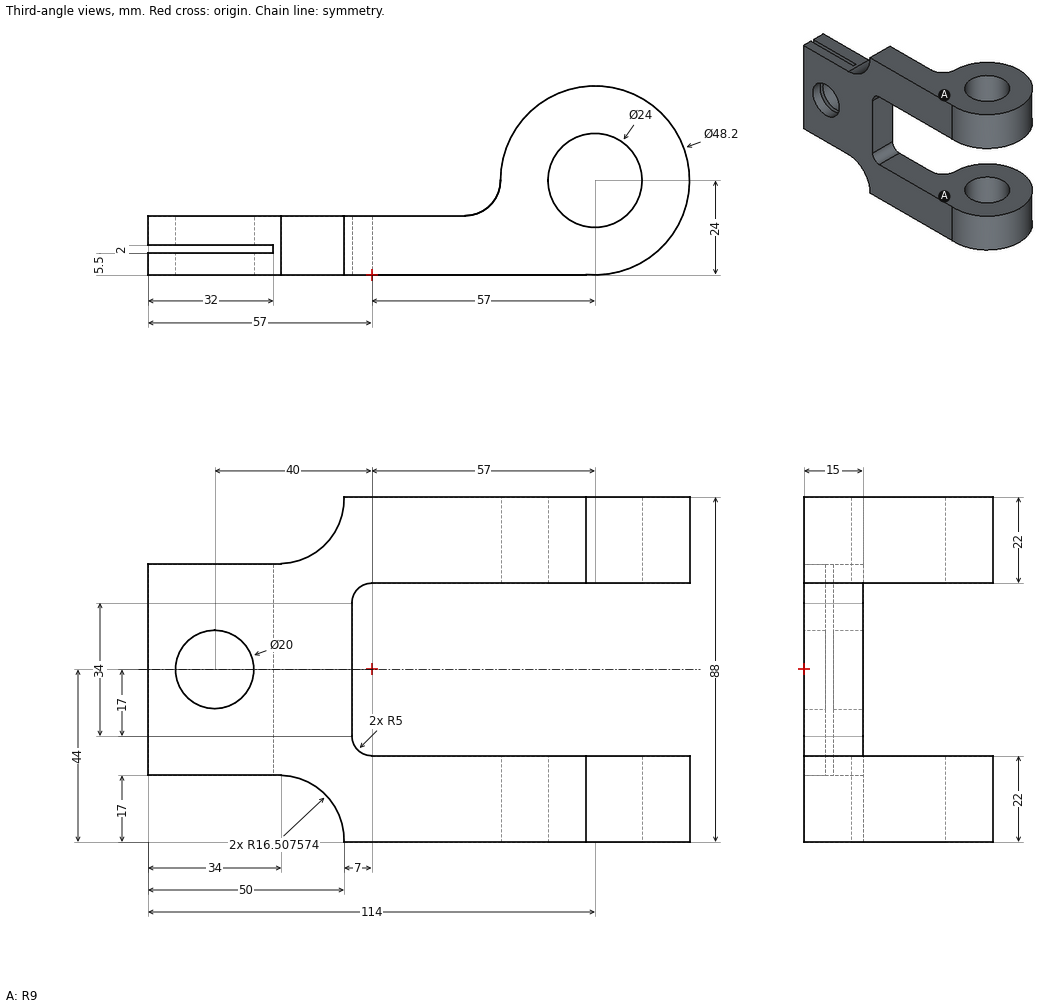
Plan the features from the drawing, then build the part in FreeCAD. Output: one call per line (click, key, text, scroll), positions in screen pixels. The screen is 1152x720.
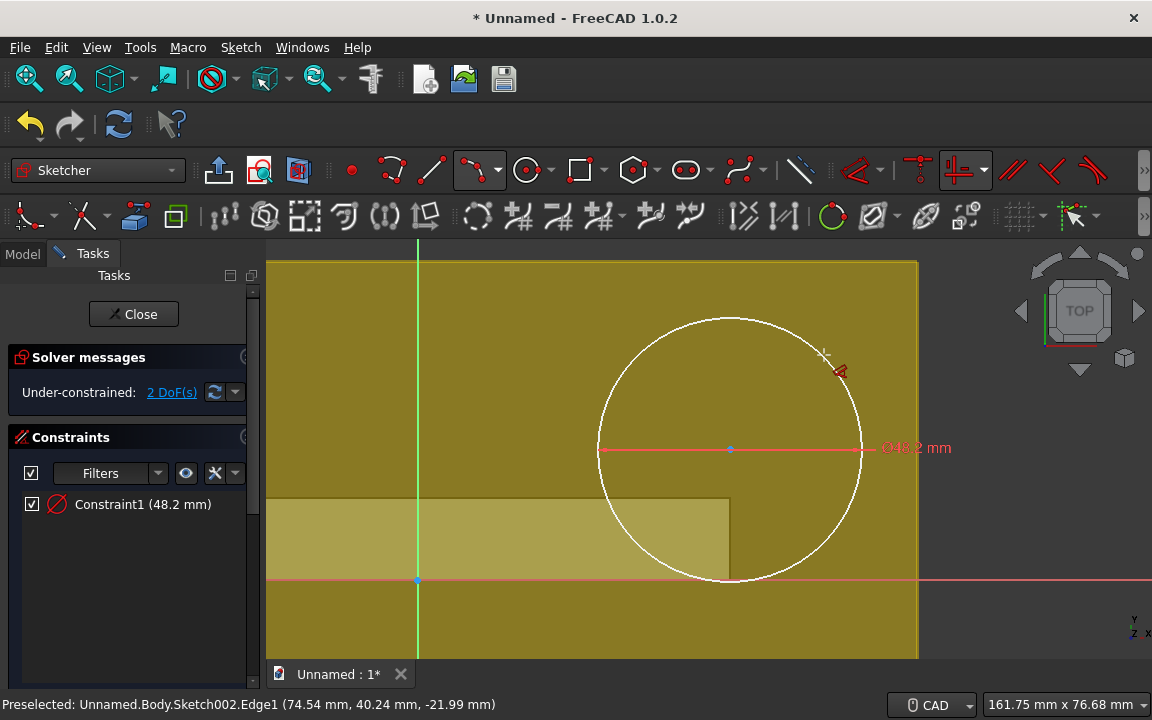
click(730, 450)
click(574, 614)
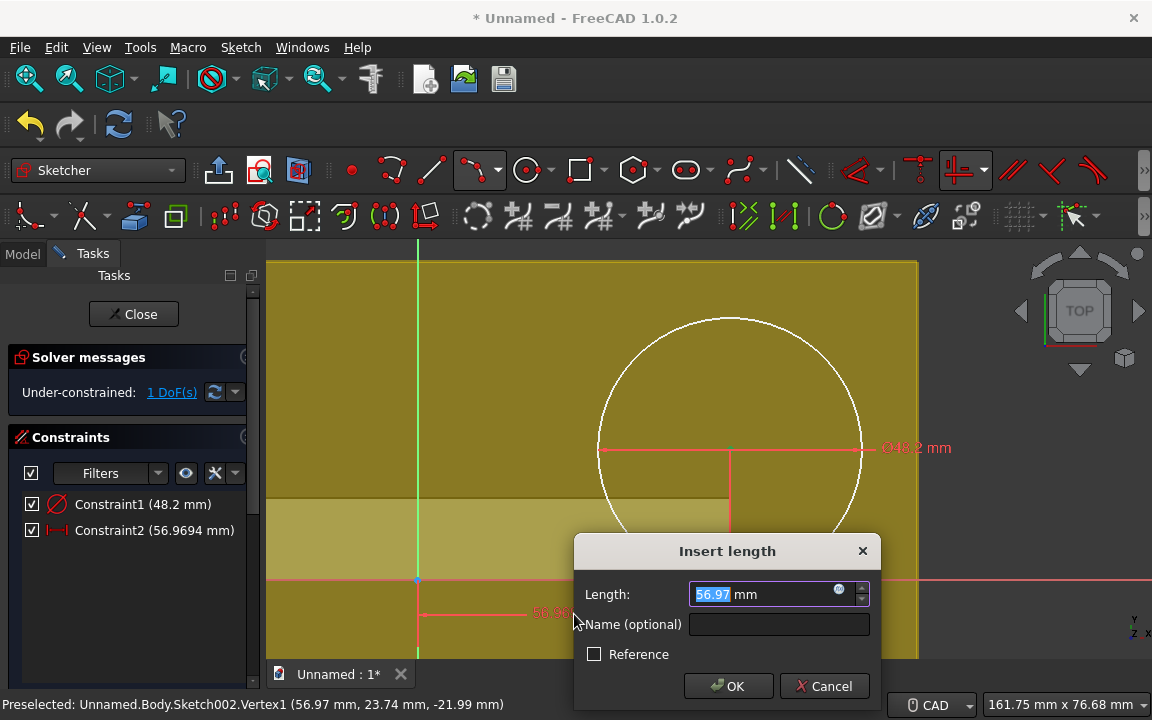
text(57)
key(Return)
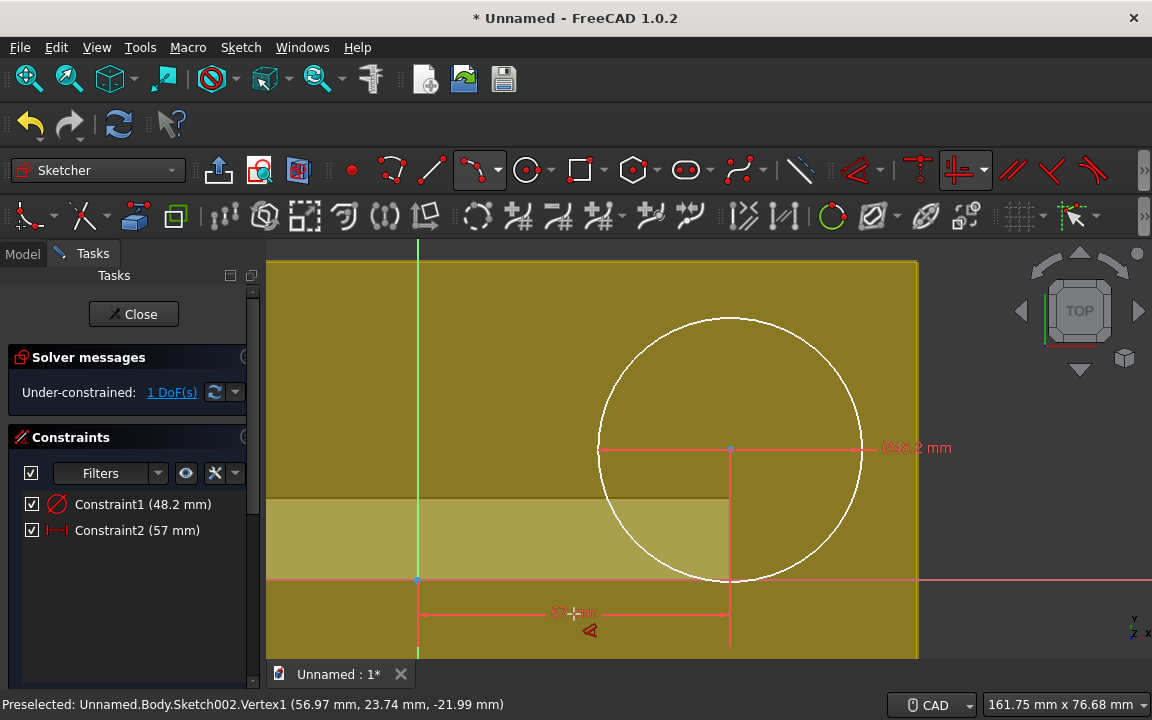
click(730, 450)
click(384, 515)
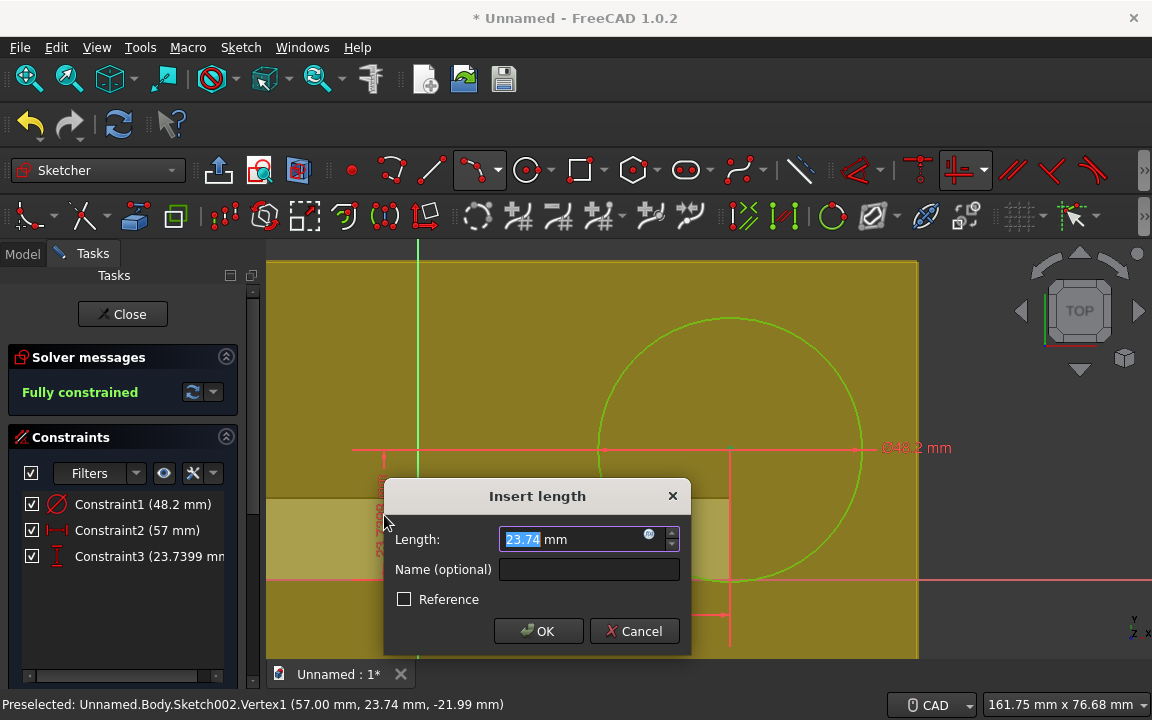
text(24)
key(Return)
key(Escape)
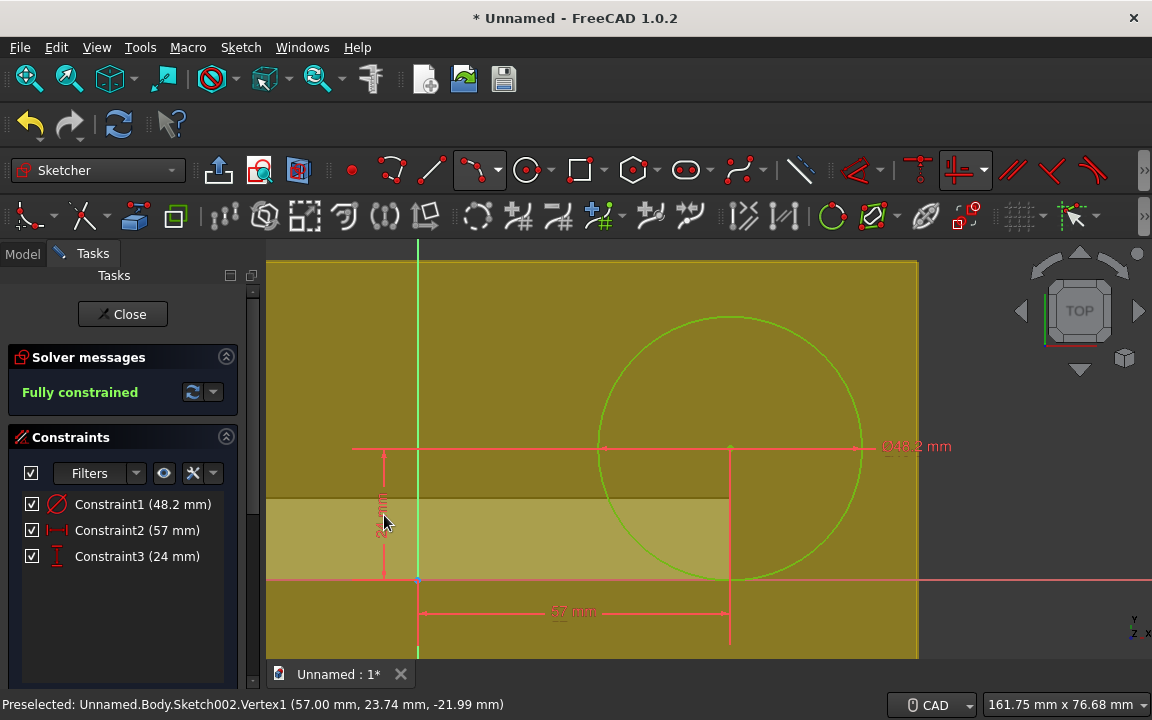
click(123, 314)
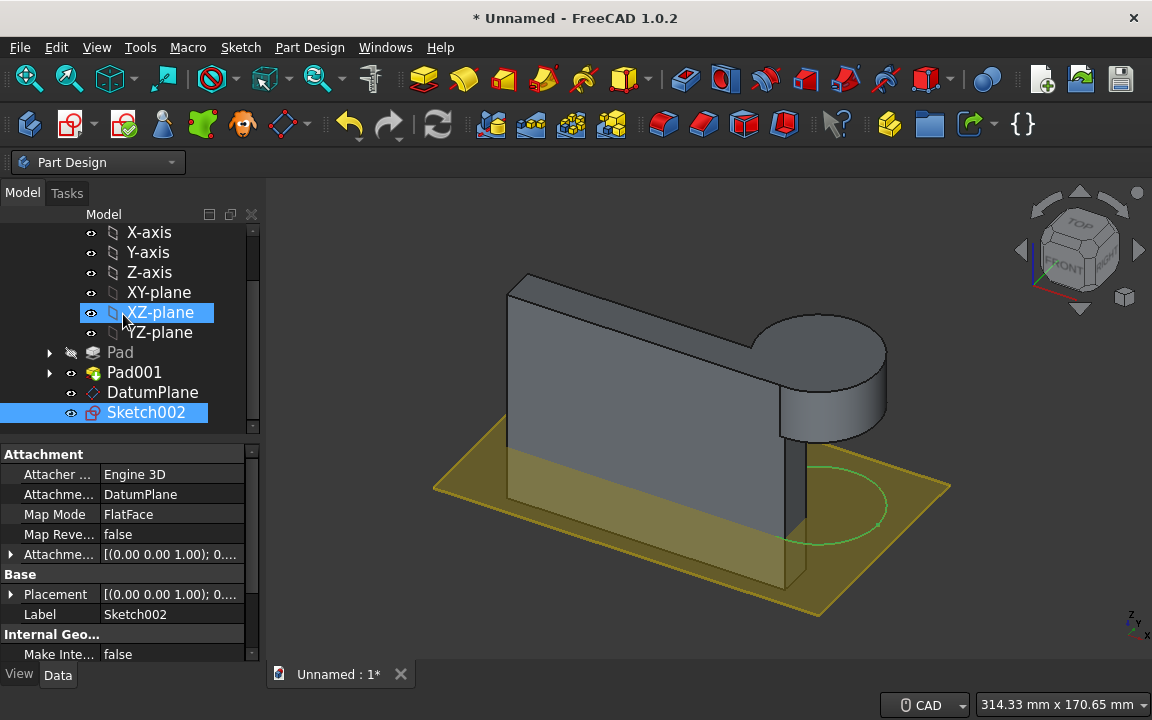
click(424, 80)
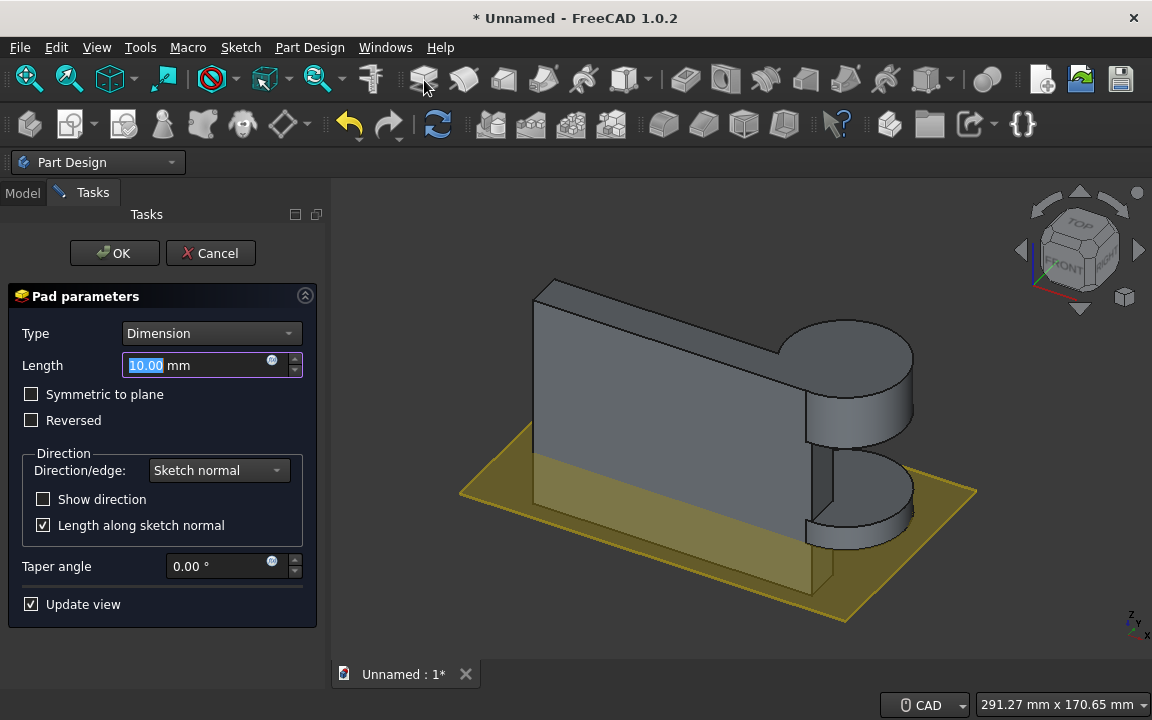
text(22)
key(Tab)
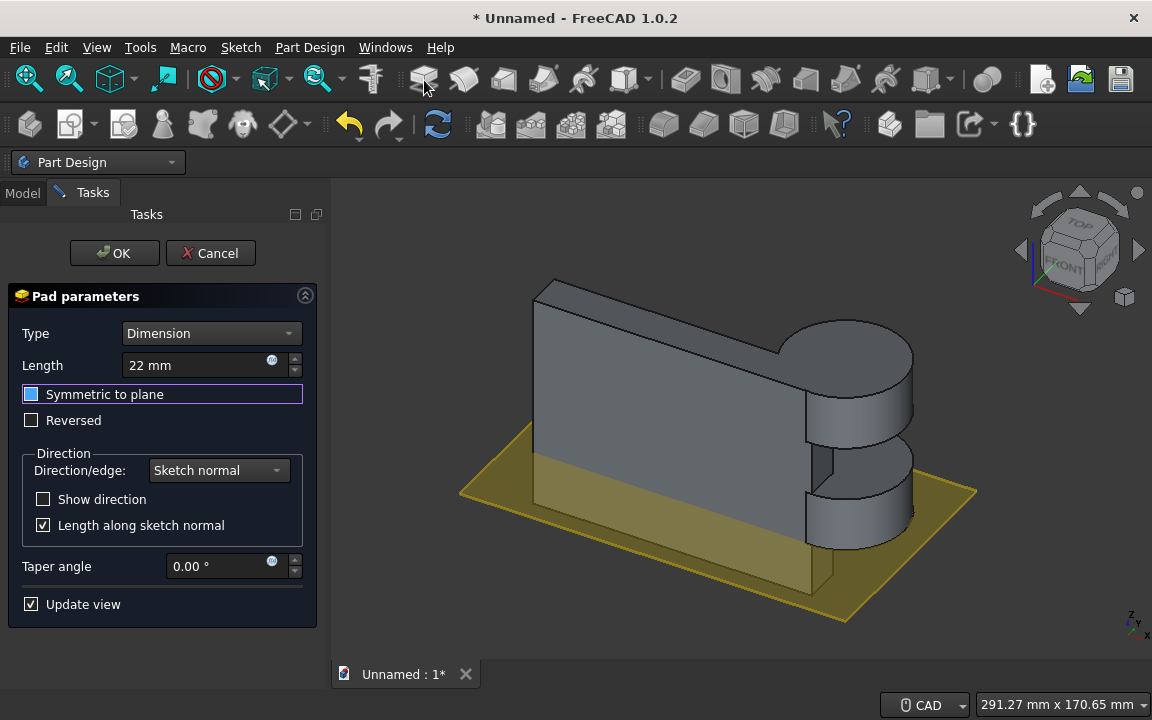
click(30, 420)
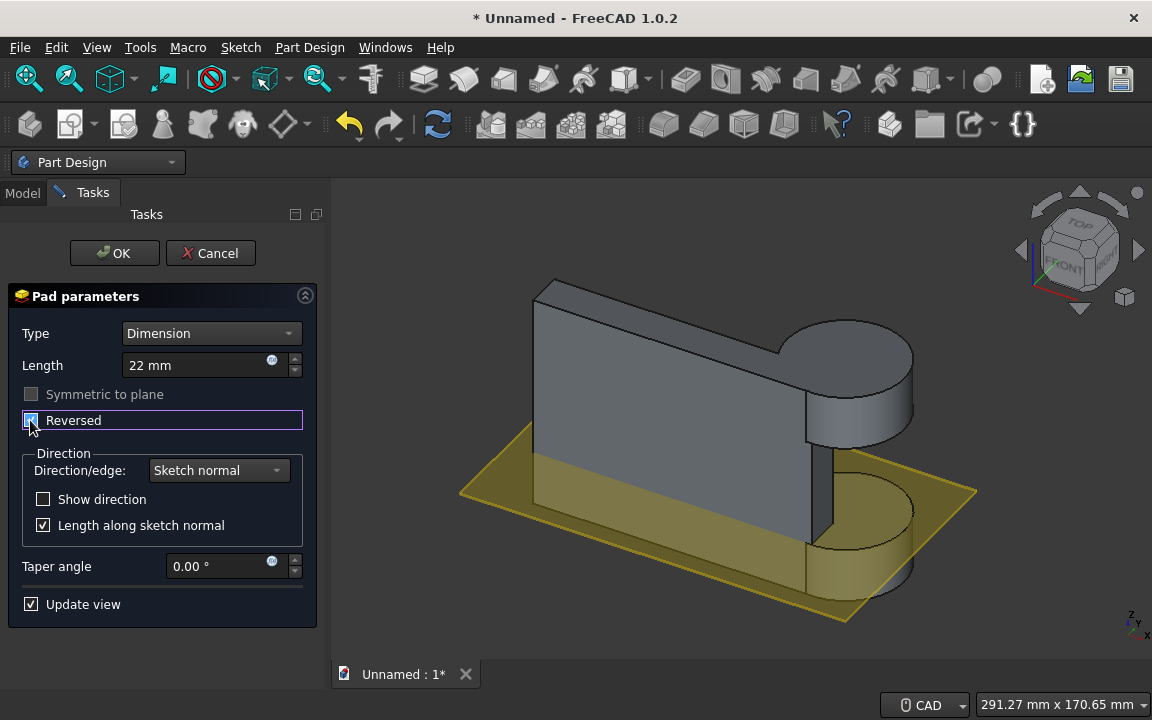
click(115, 253)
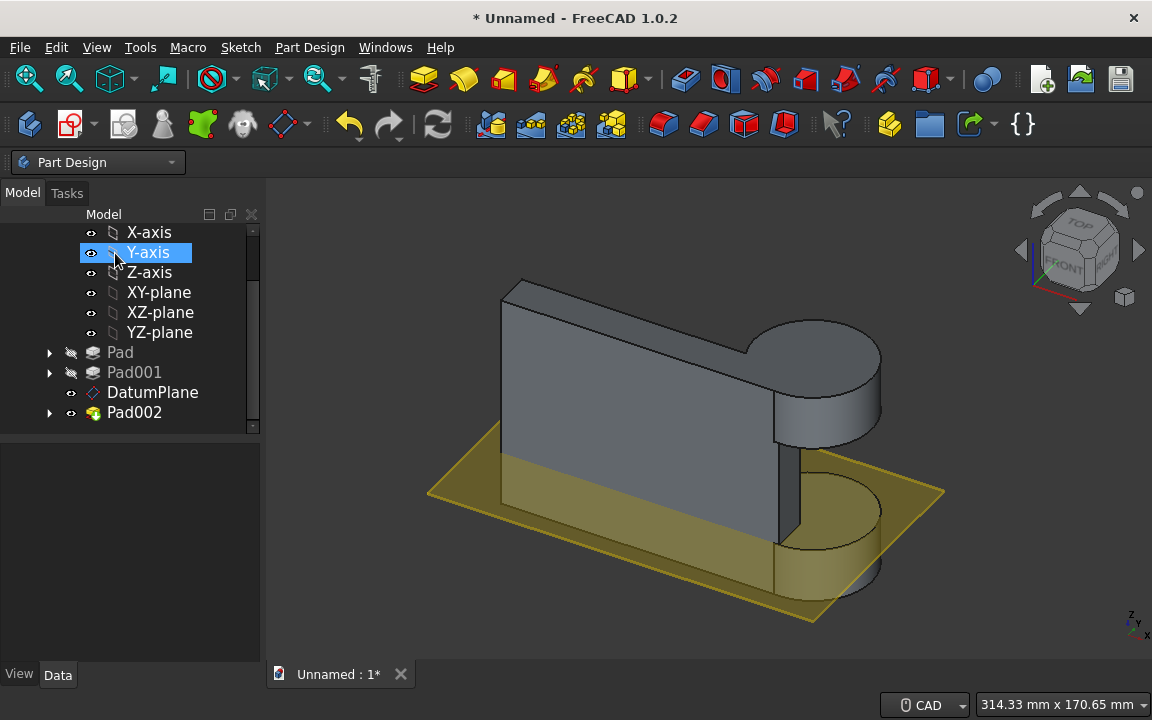
click(116, 393)
key(space)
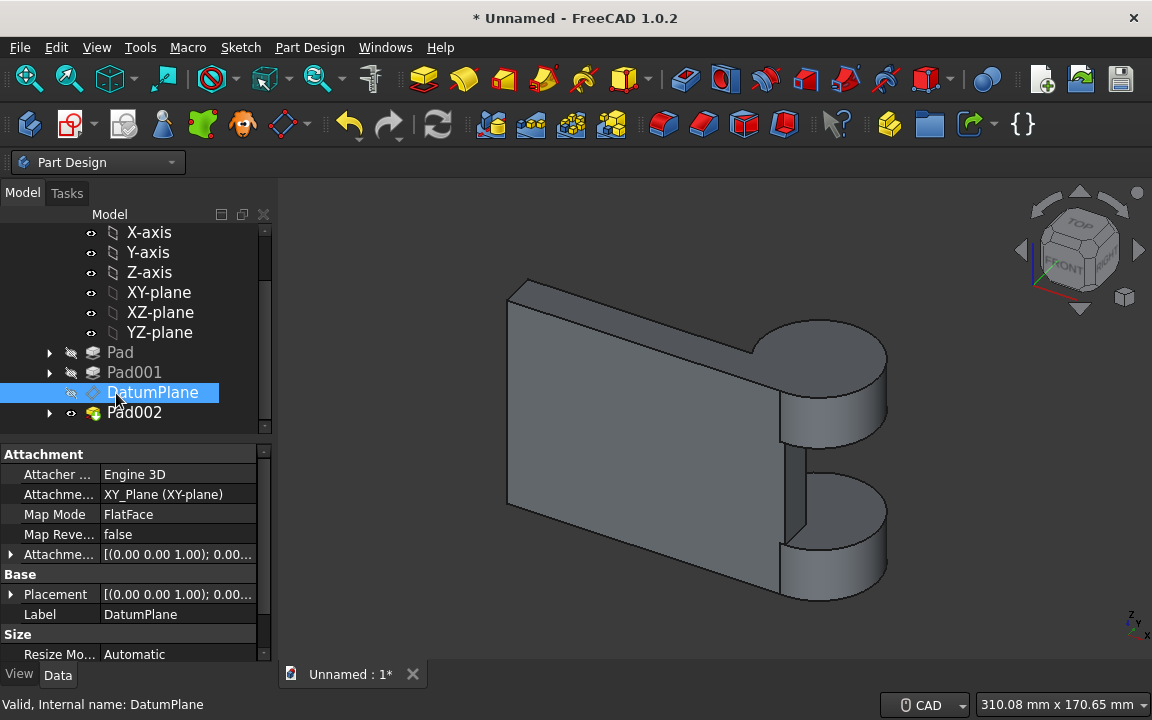
key(5)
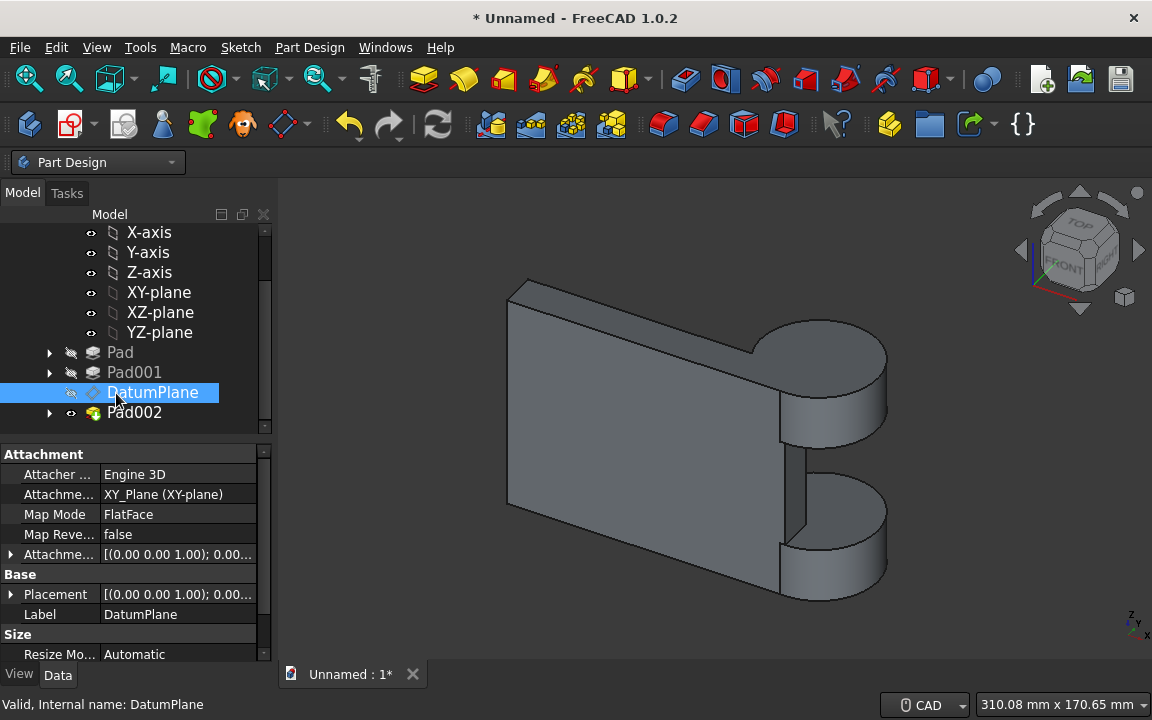
key(v)
key(f)